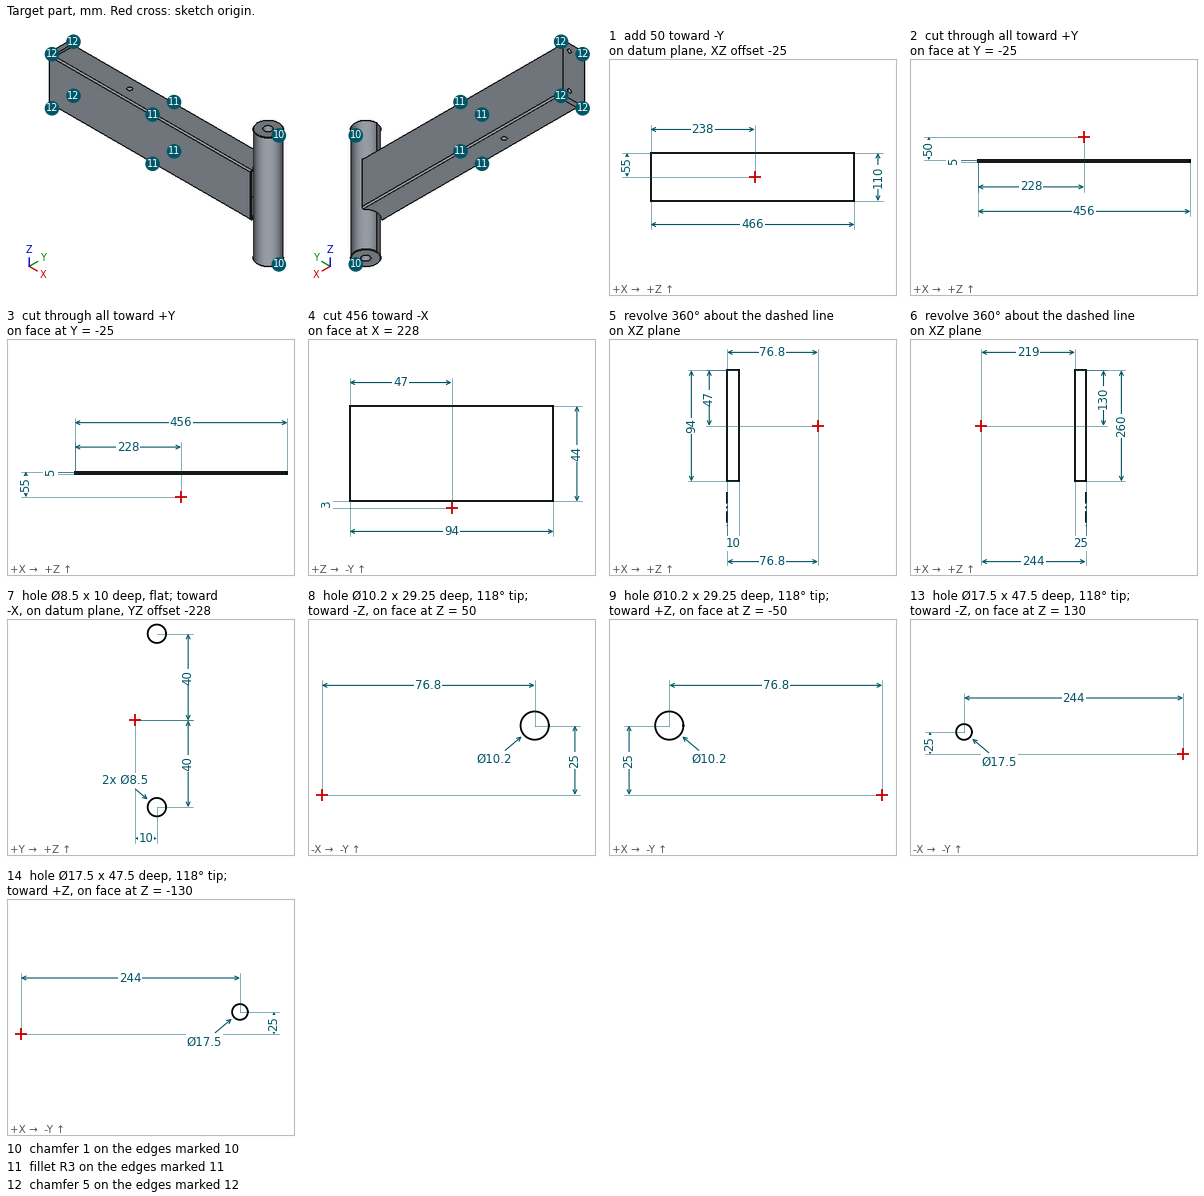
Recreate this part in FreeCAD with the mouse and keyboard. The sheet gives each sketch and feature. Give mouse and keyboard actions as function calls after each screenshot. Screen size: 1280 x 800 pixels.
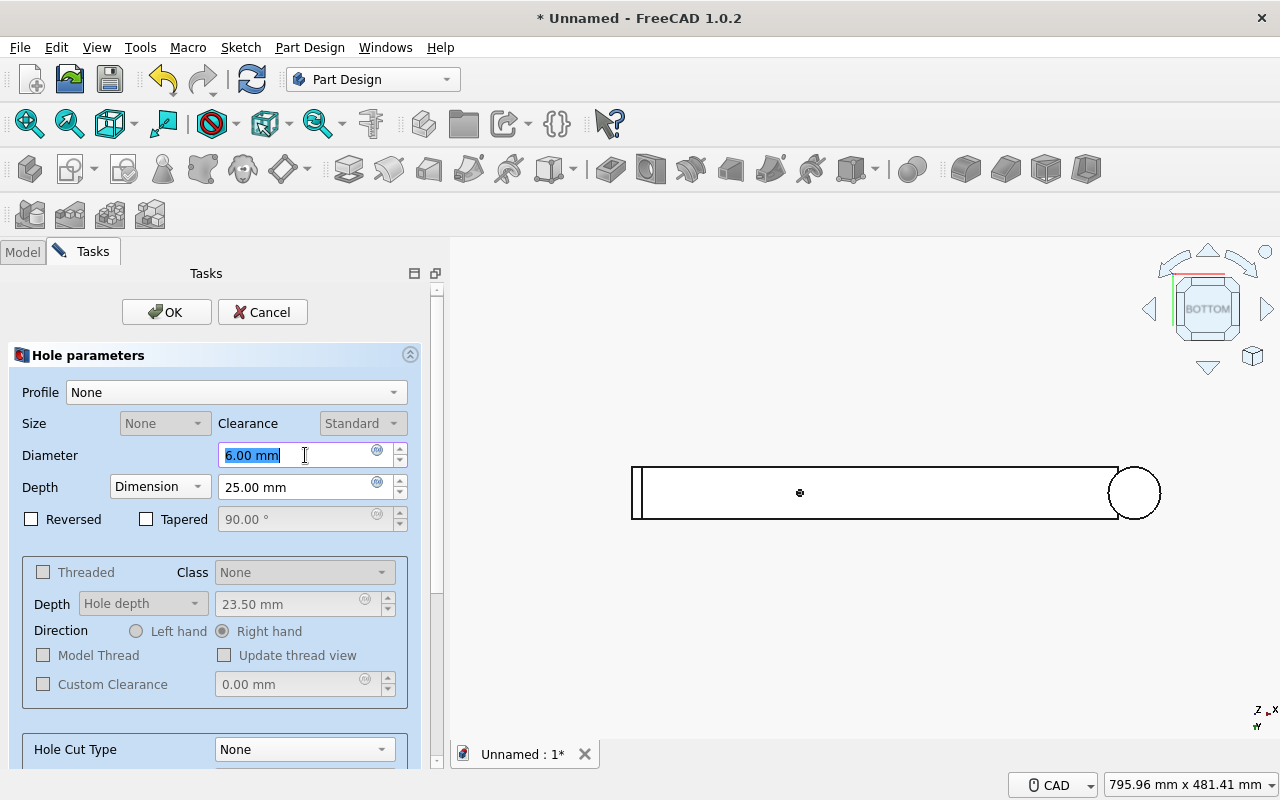
text(10.2)
key(Tab)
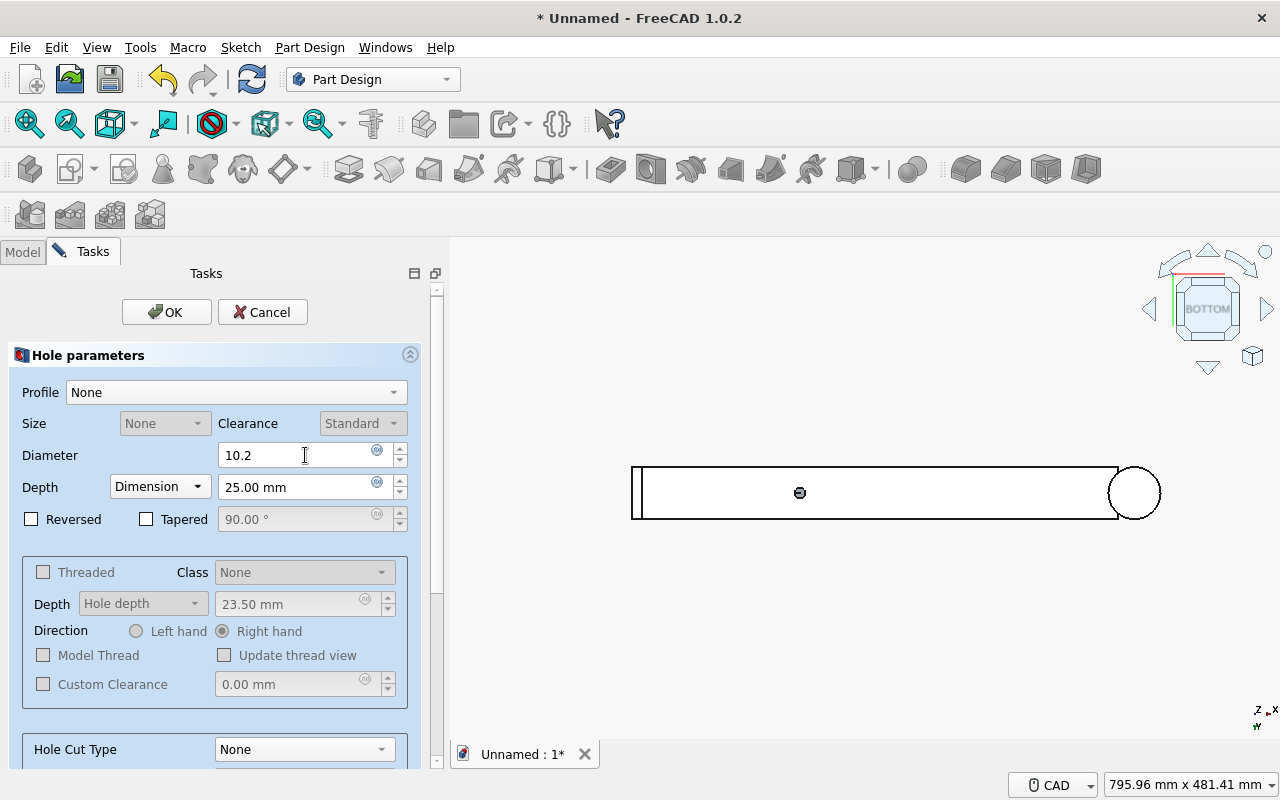
triple_click(305, 487)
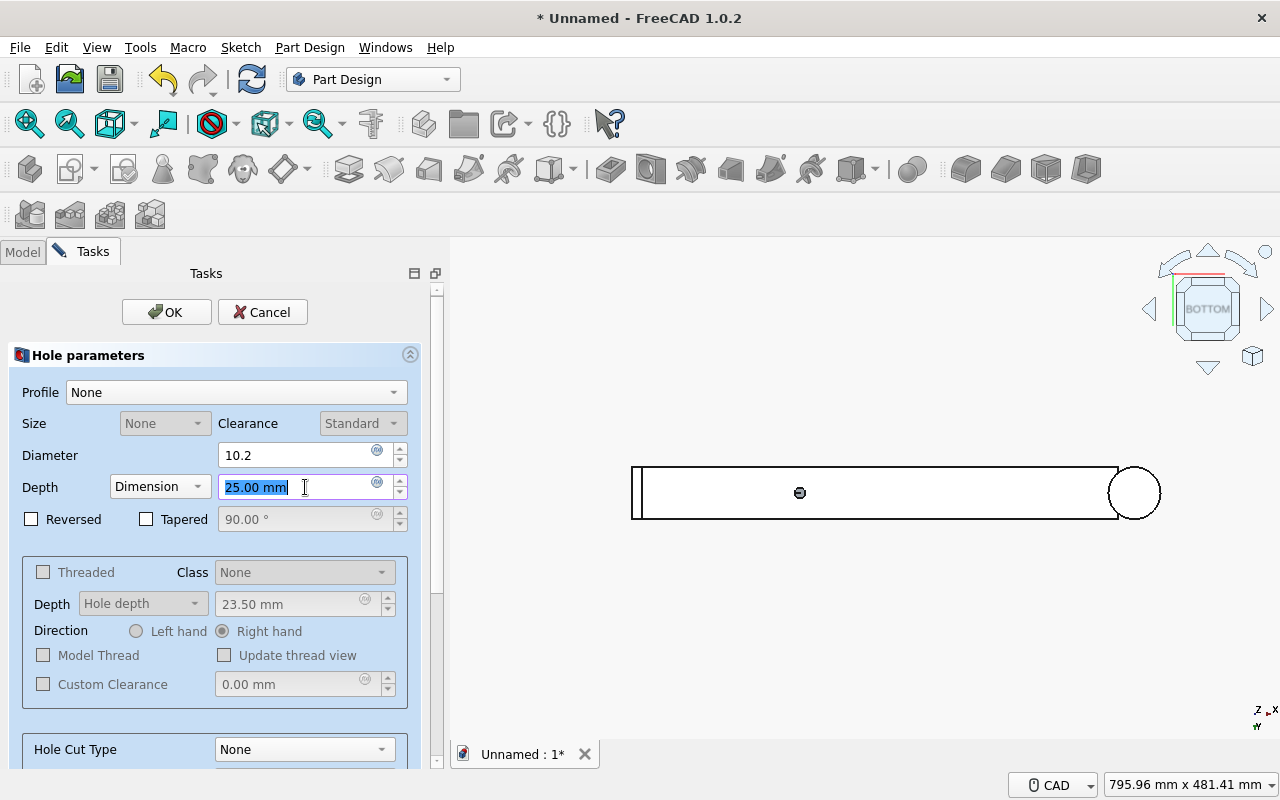
text(29.25)
key(Tab)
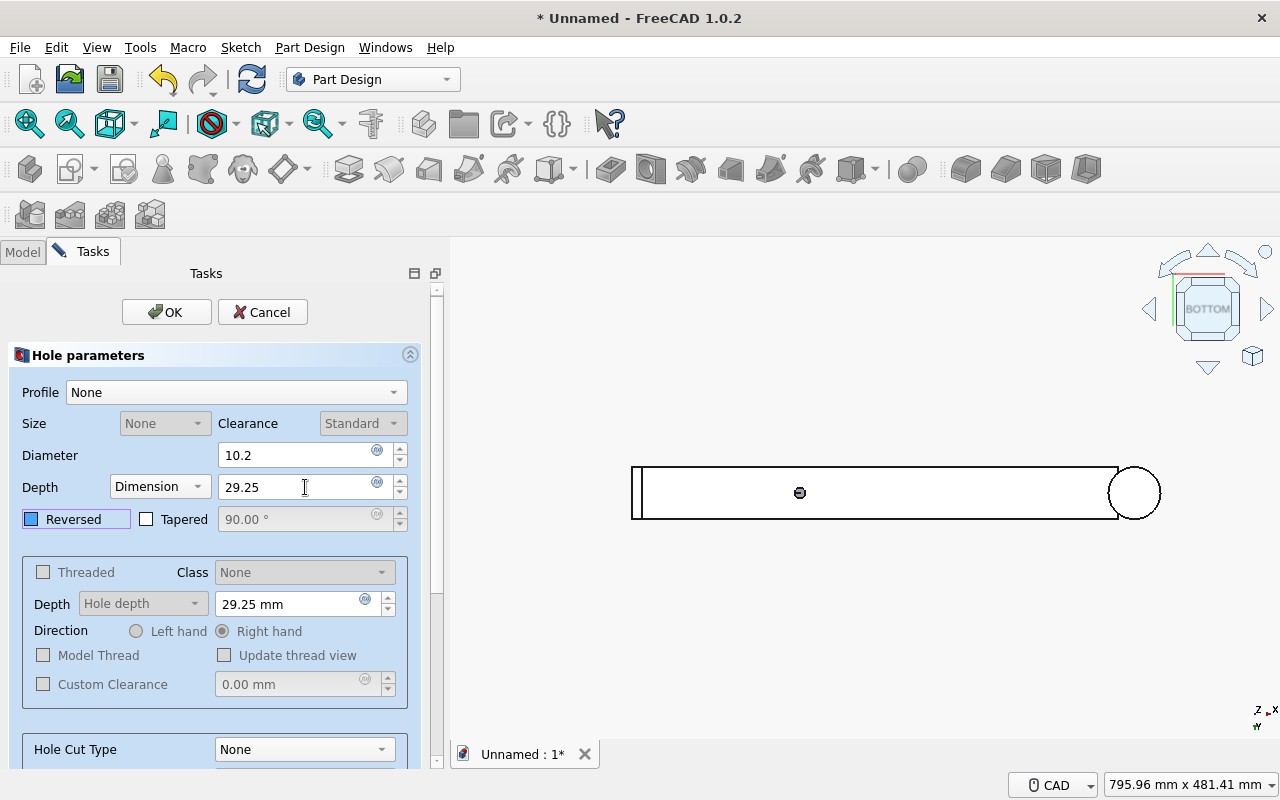
click(167, 312)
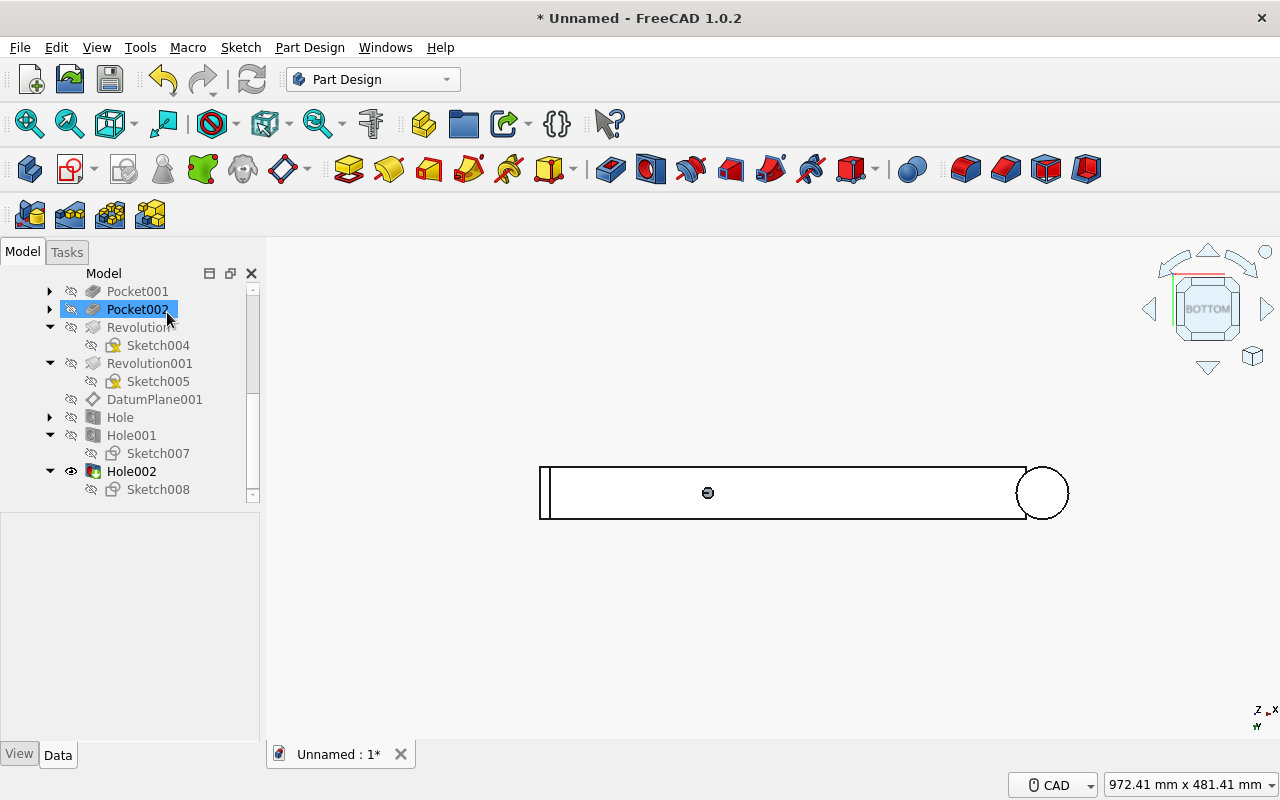
click(1069, 492)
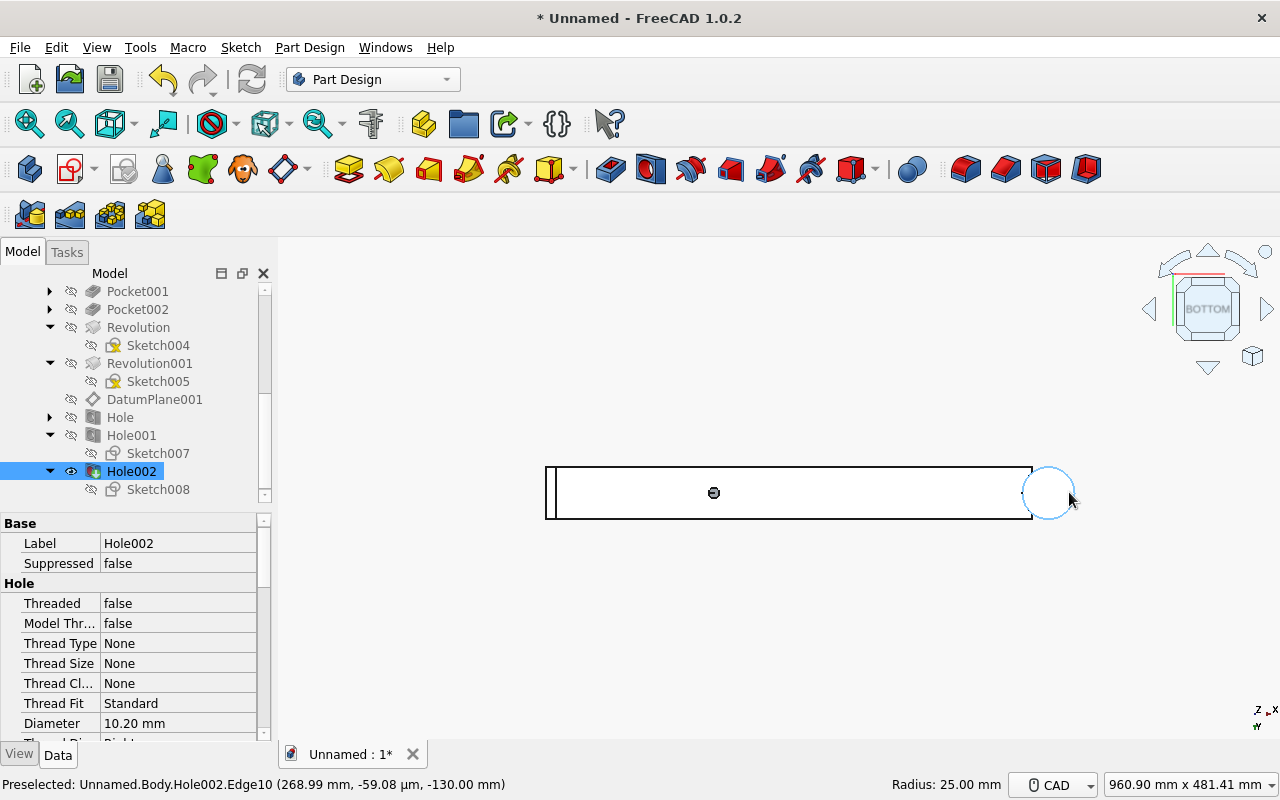
key(0)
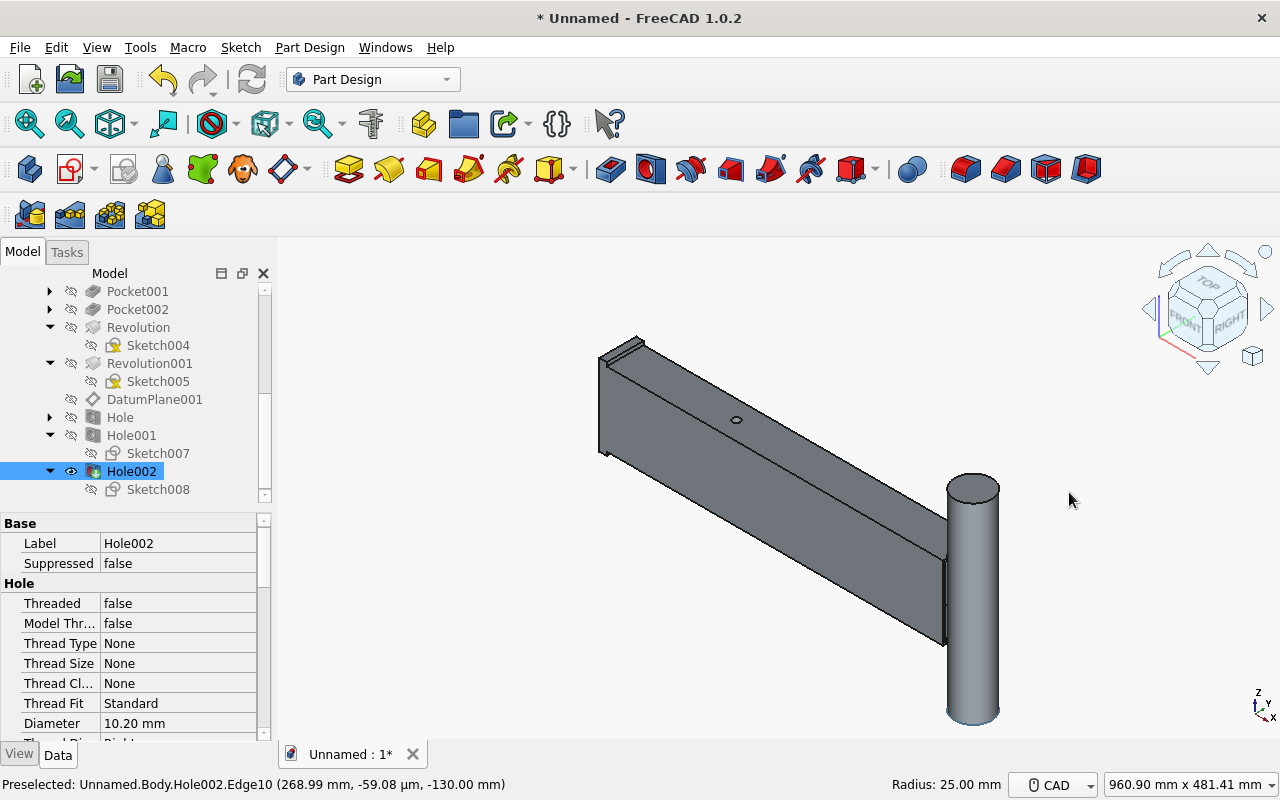
click(992, 498, ctrl)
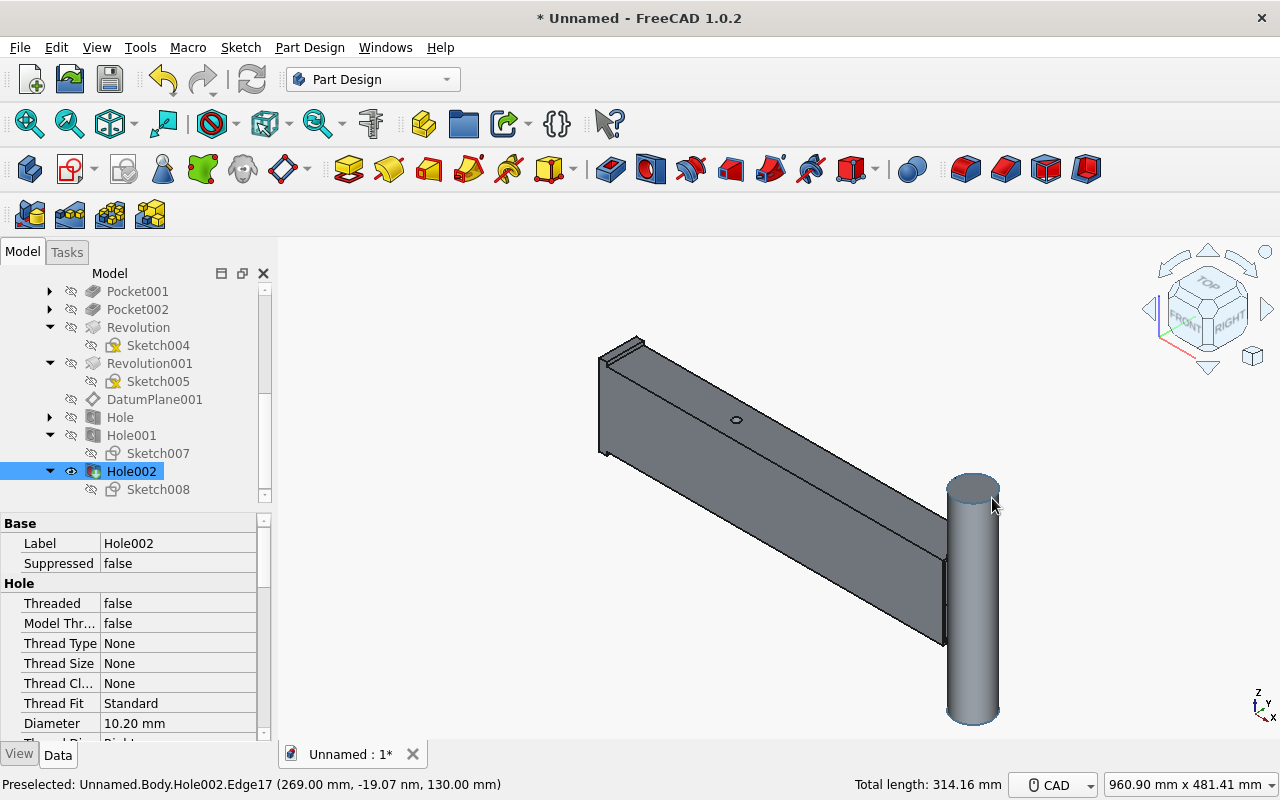
click(1006, 170)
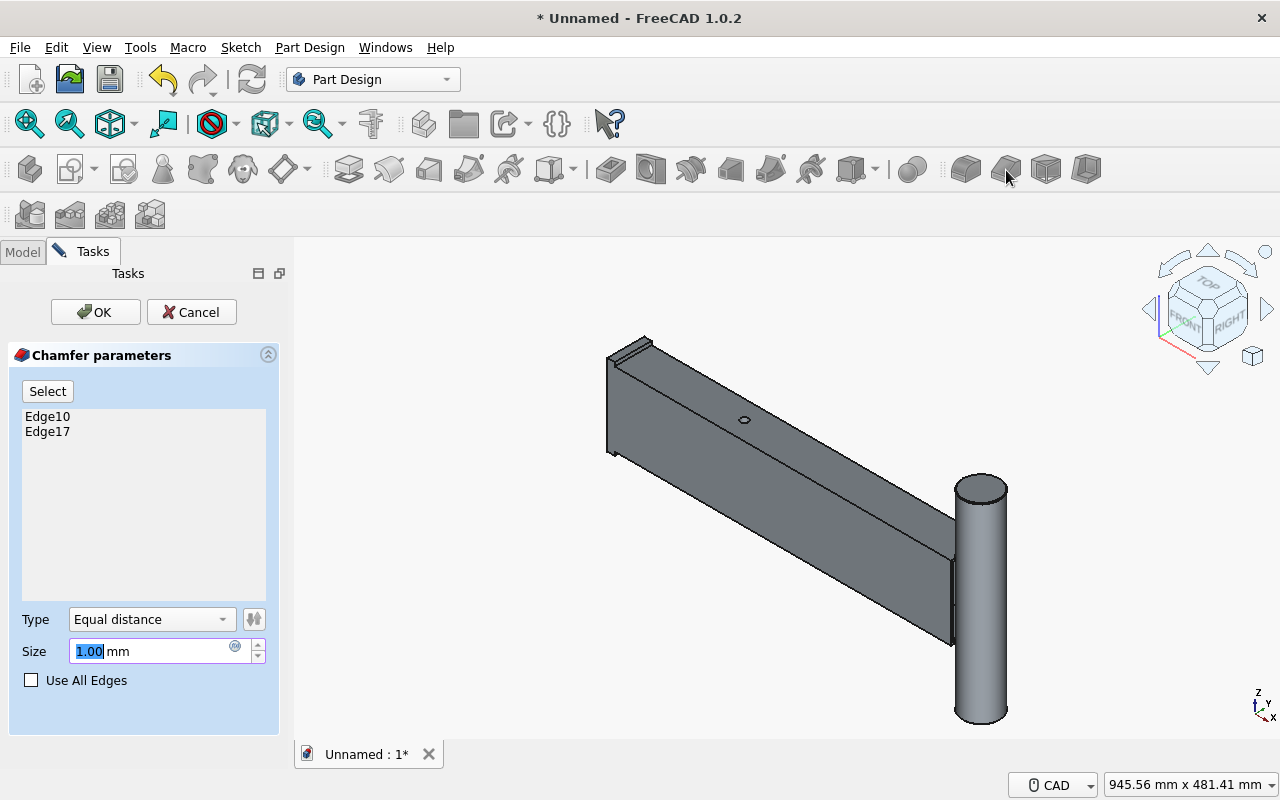
text(1)
key(Tab)